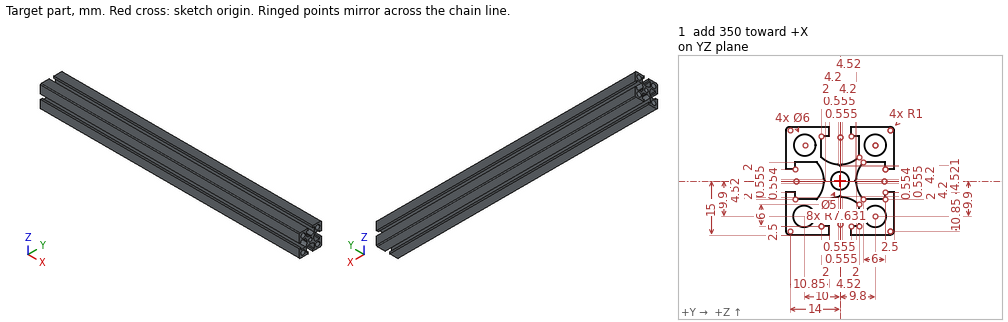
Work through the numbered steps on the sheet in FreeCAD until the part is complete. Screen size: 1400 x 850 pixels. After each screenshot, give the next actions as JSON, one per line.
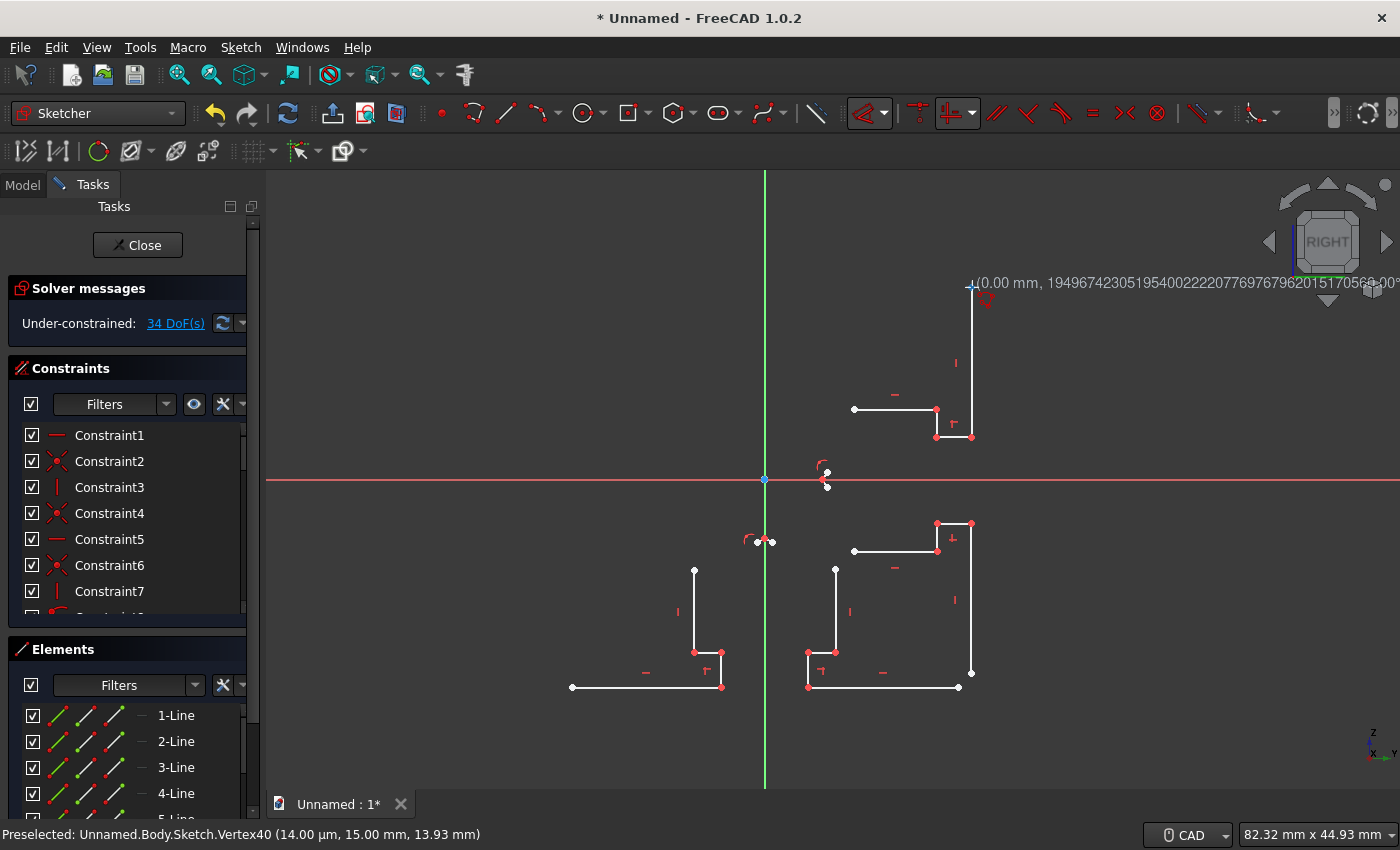
{"action": "left_click", "coordinate": [958, 273]}
{"action": "left_click", "coordinate": [808, 273]}
{"action": "left_click", "coordinate": [808, 308]}
{"action": "left_click", "coordinate": [836, 308]}
{"action": "left_click", "coordinate": [836, 390]}
{"action": "right_click", "coordinate": [836, 390]}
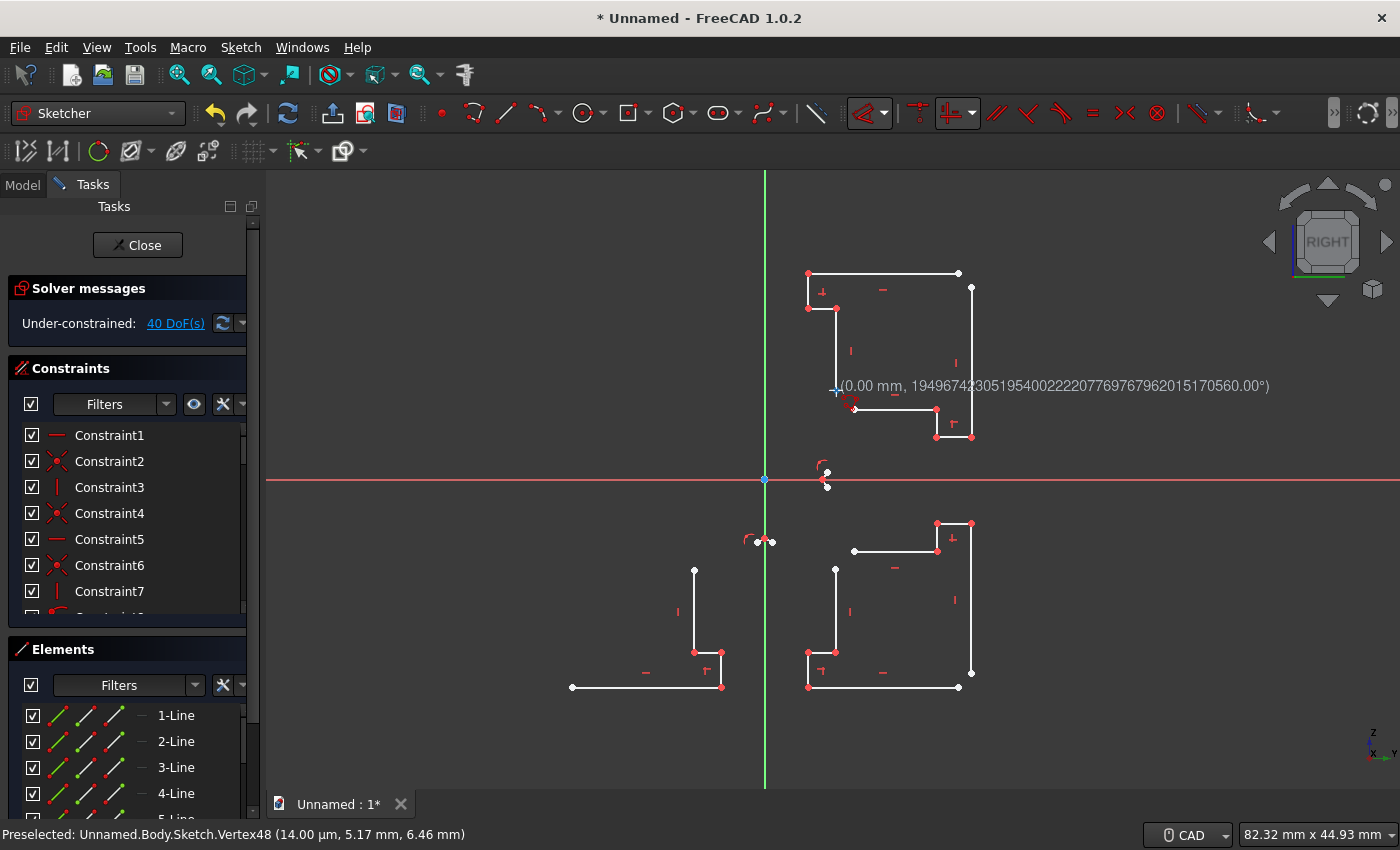
{"action": "scroll", "coordinate": [772, 418], "scroll_direction": "up", "scroll_amount": 4}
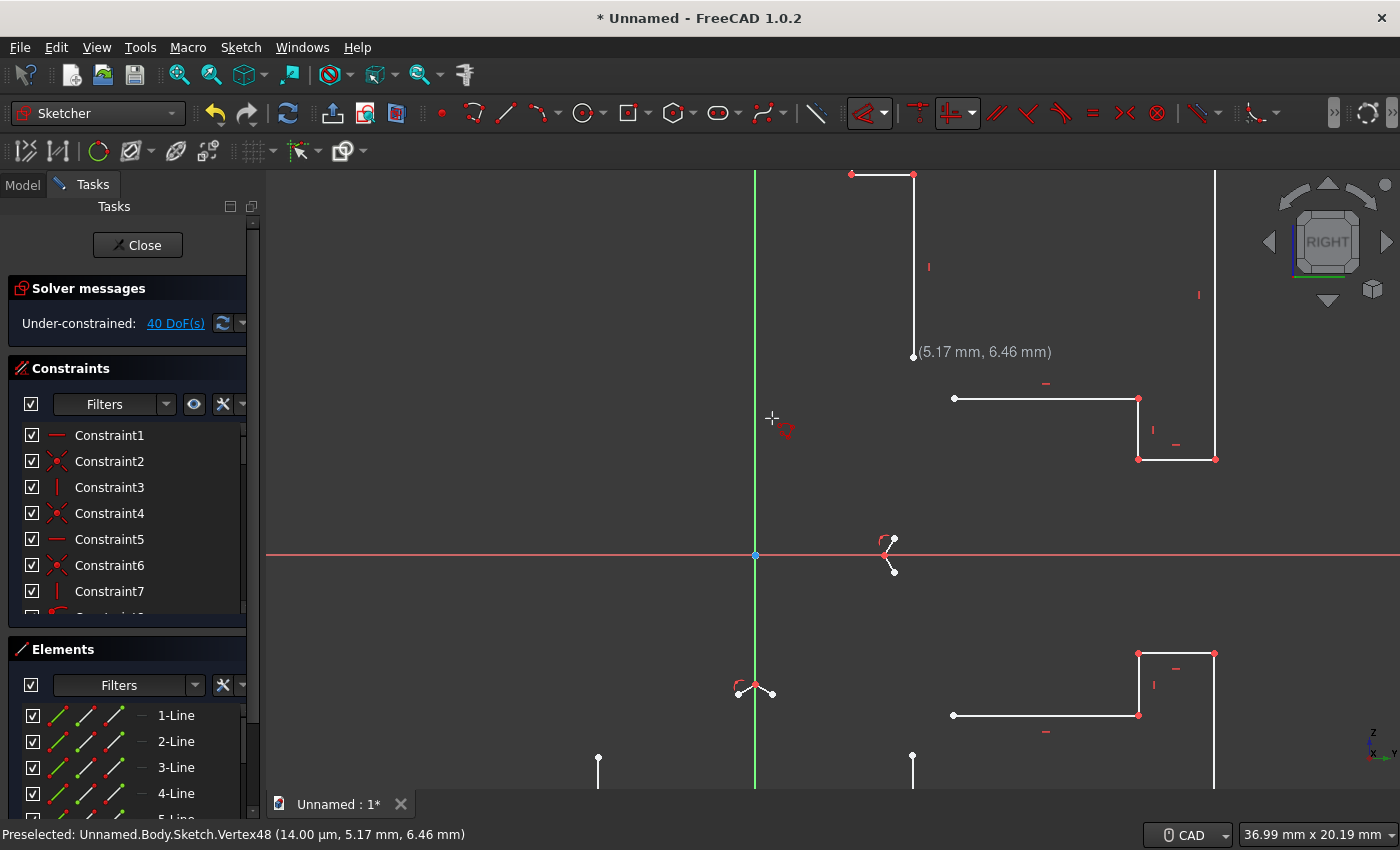
{"action": "left_click", "coordinate": [772, 417]}
{"action": "left_click", "coordinate": [755, 427]}
{"action": "left_click", "coordinate": [738, 417]}
{"action": "right_click", "coordinate": [738, 417]}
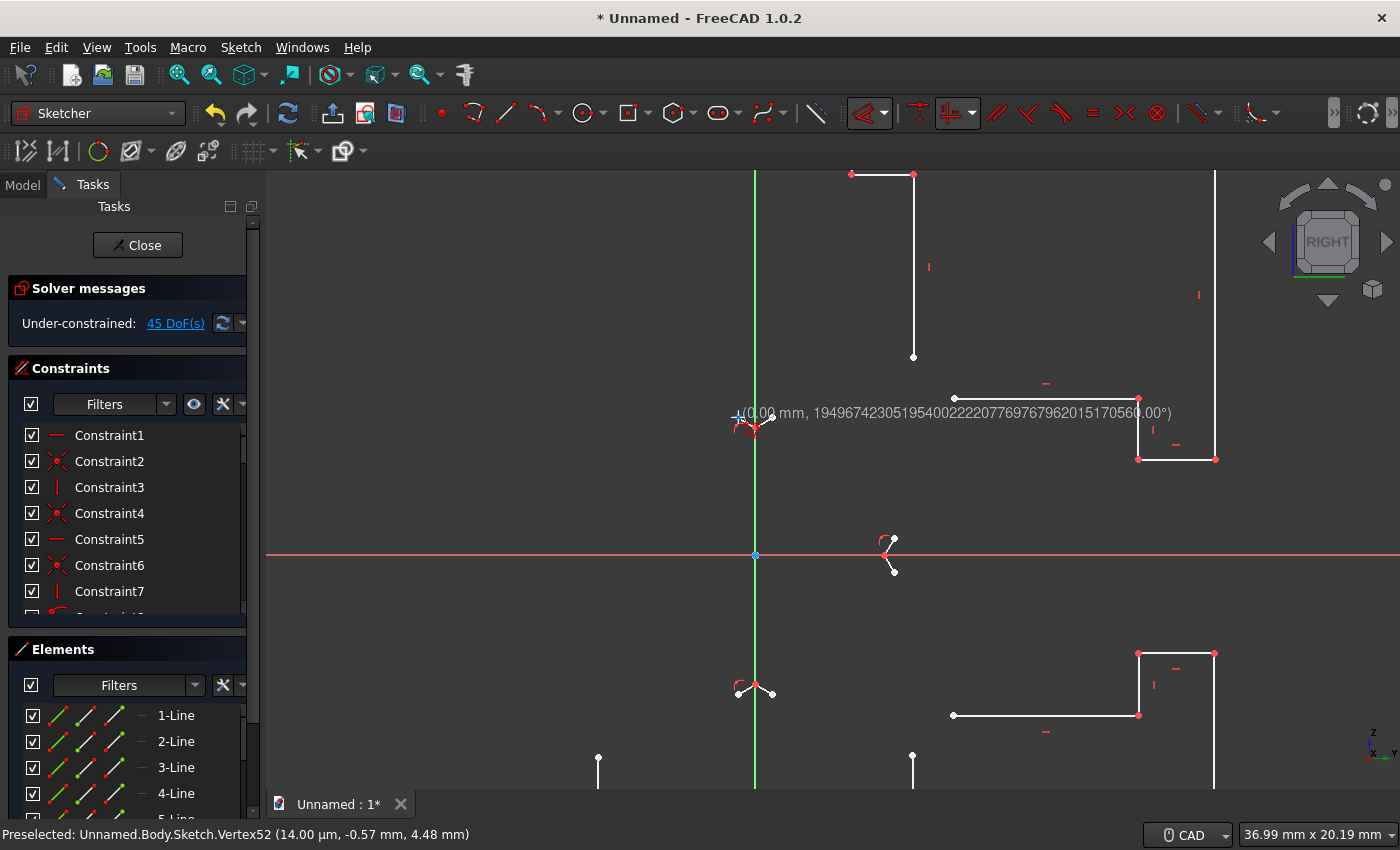
{"action": "left_click", "coordinate": [598, 356]}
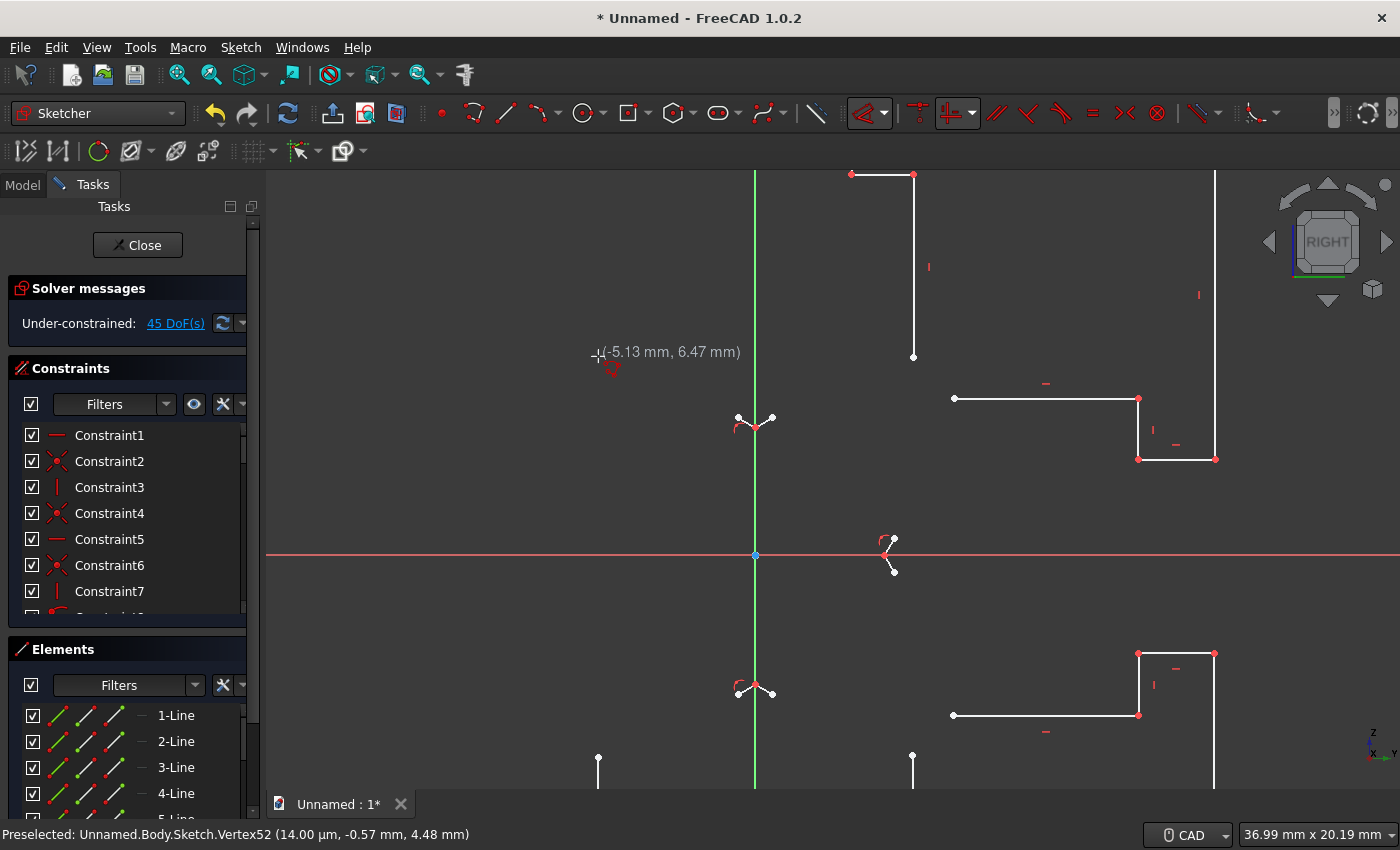
{"action": "scroll", "coordinate": [772, 418], "scroll_direction": "down", "scroll_amount": 4}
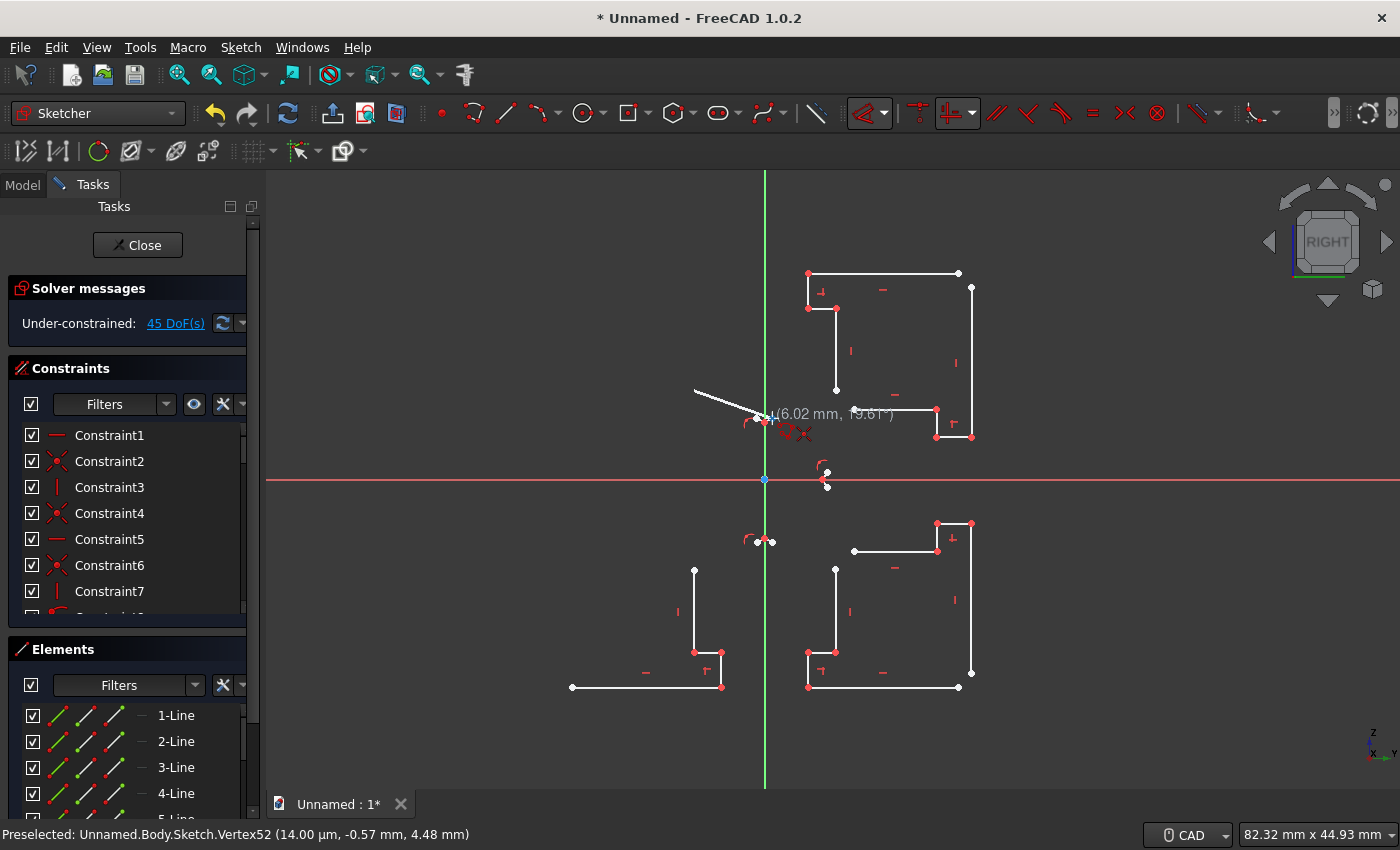
{"action": "left_click", "coordinate": [694, 308]}
{"action": "left_click", "coordinate": [721, 308]}
{"action": "left_click", "coordinate": [721, 273]}
{"action": "left_click", "coordinate": [572, 273]}
{"action": "right_click", "coordinate": [572, 273]}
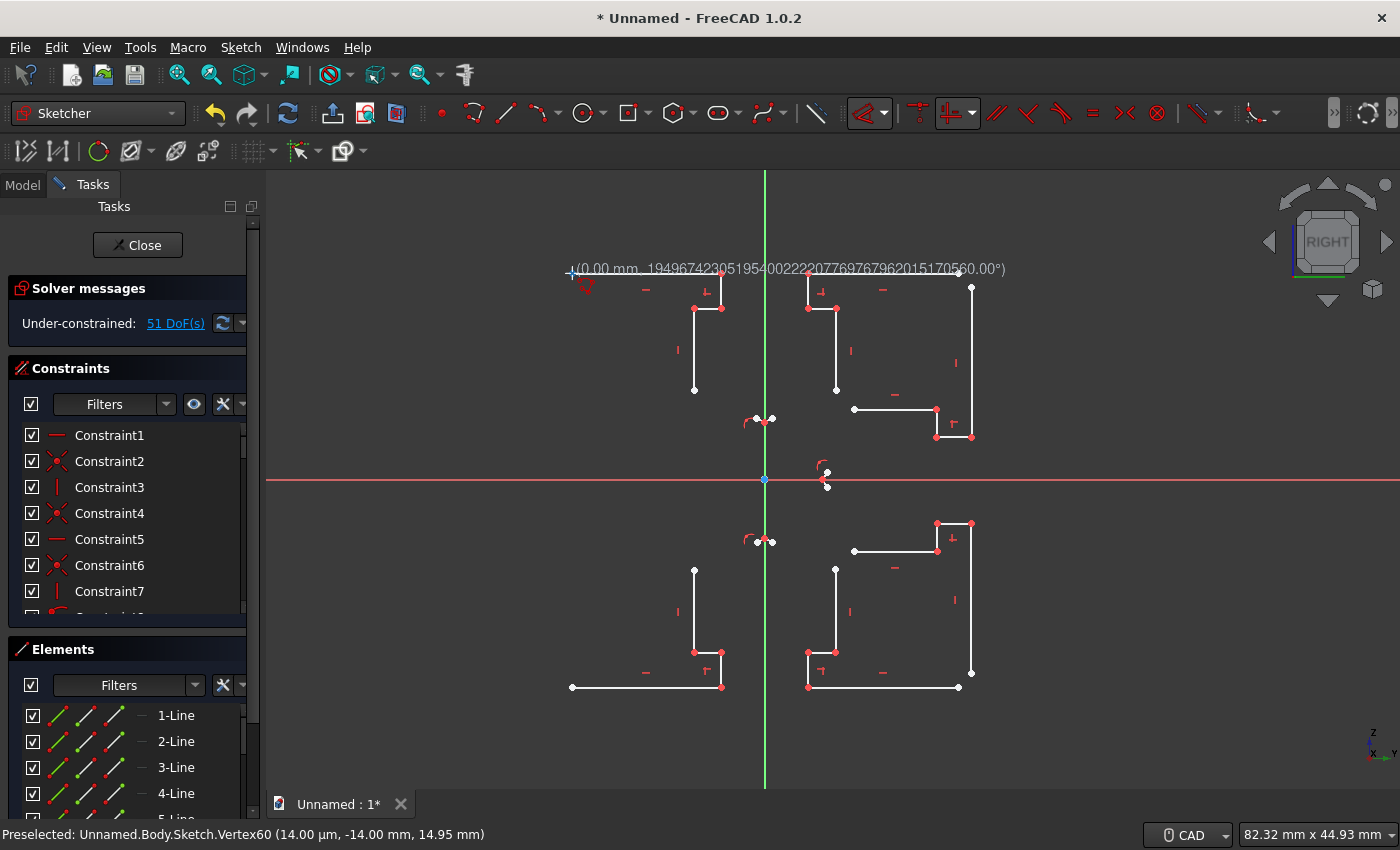
{"action": "left_click", "coordinate": [558, 287]}
{"action": "left_click", "coordinate": [558, 437]}
{"action": "left_click", "coordinate": [593, 437]}
{"action": "left_click", "coordinate": [593, 409]}
{"action": "left_click", "coordinate": [675, 409]}
{"action": "right_click", "coordinate": [675, 409]}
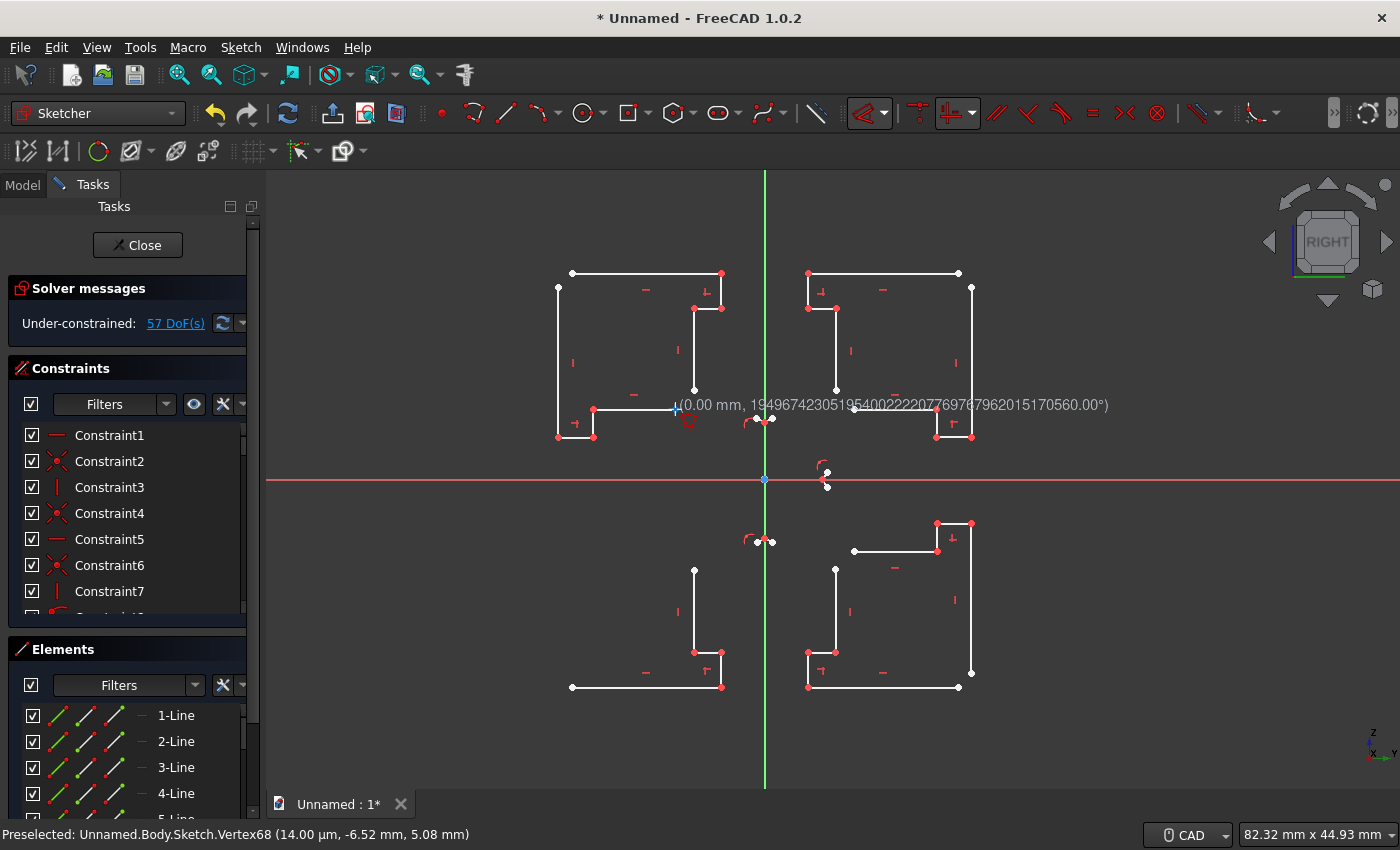
{"action": "scroll", "coordinate": [703, 472], "scroll_direction": "up", "scroll_amount": 4}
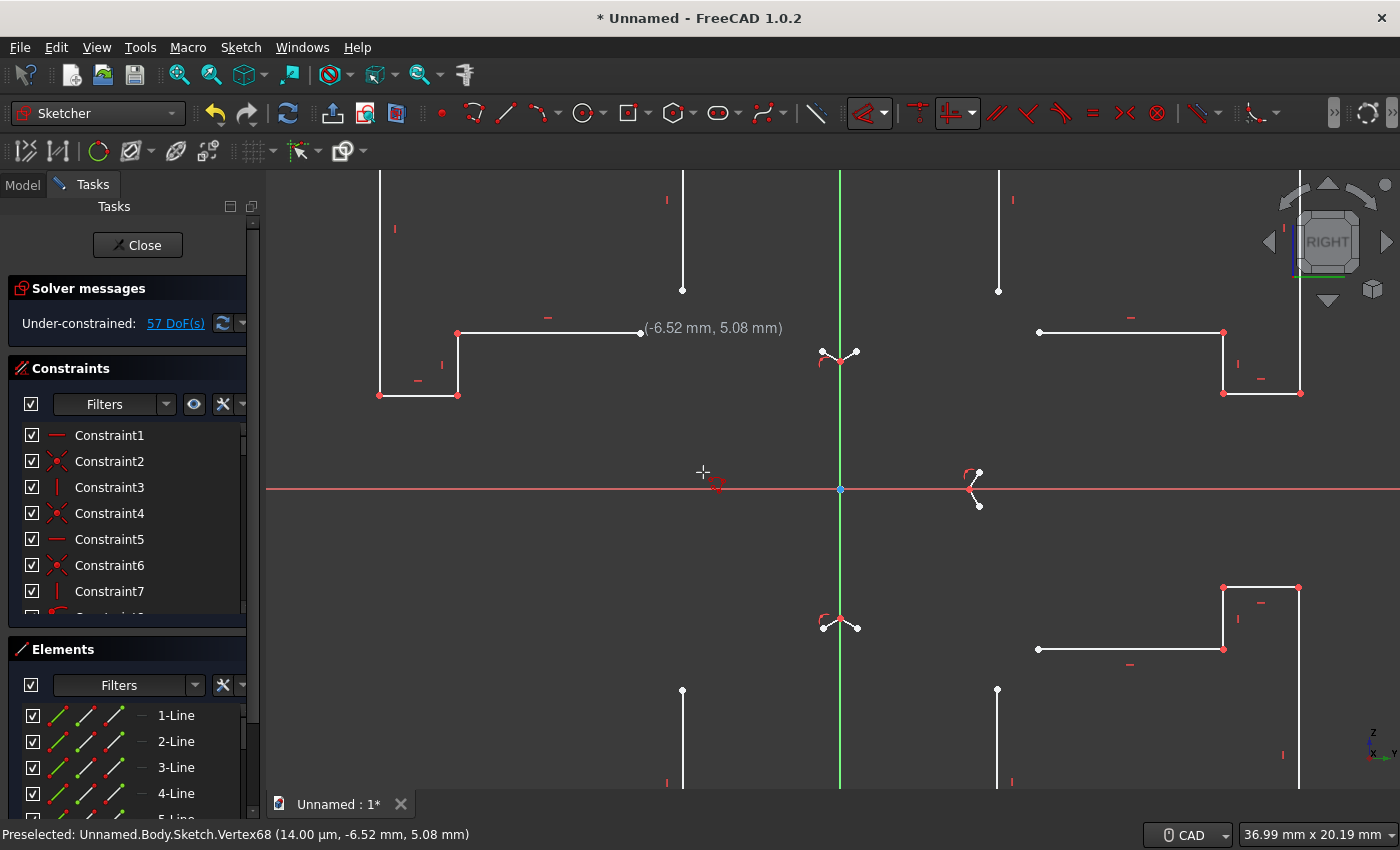
{"action": "left_click", "coordinate": [701, 472]}
{"action": "left_click", "coordinate": [711, 489]}
{"action": "left_click", "coordinate": [701, 506]}
{"action": "right_click", "coordinate": [701, 506]}